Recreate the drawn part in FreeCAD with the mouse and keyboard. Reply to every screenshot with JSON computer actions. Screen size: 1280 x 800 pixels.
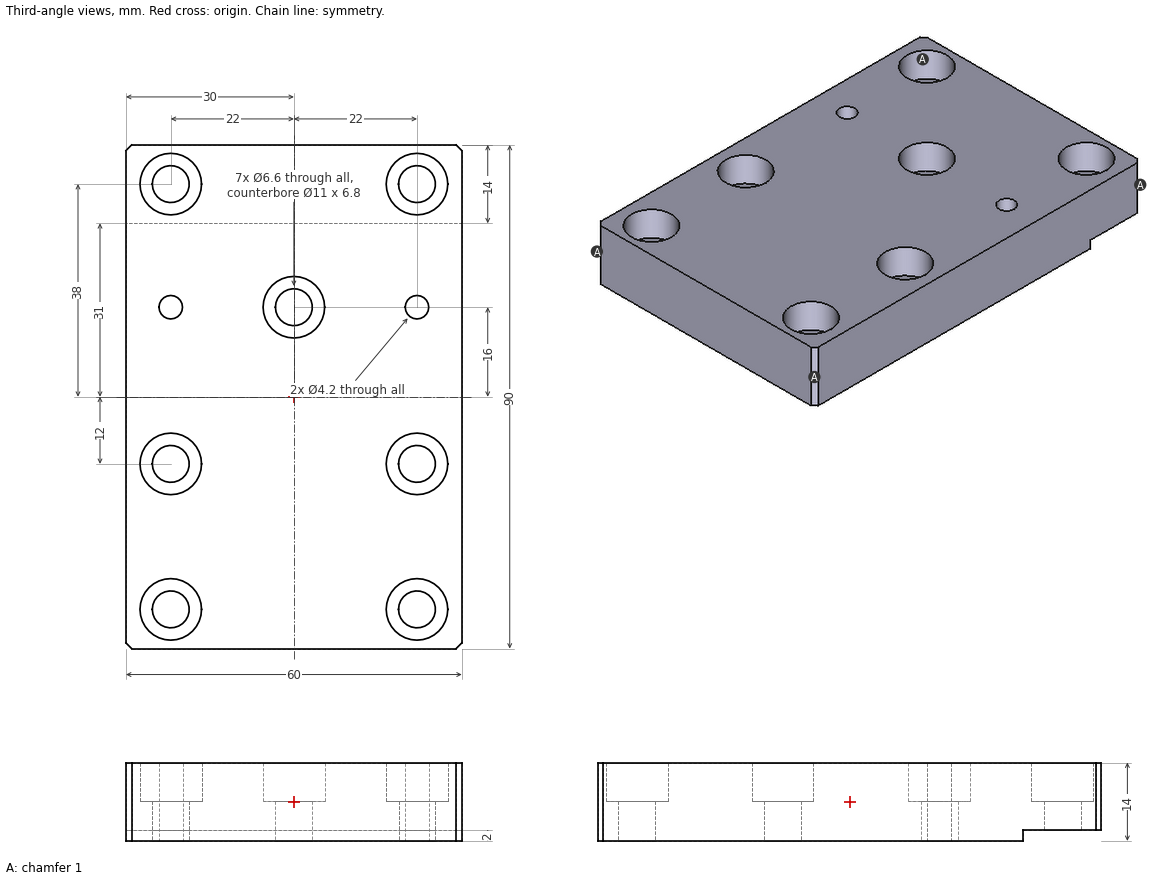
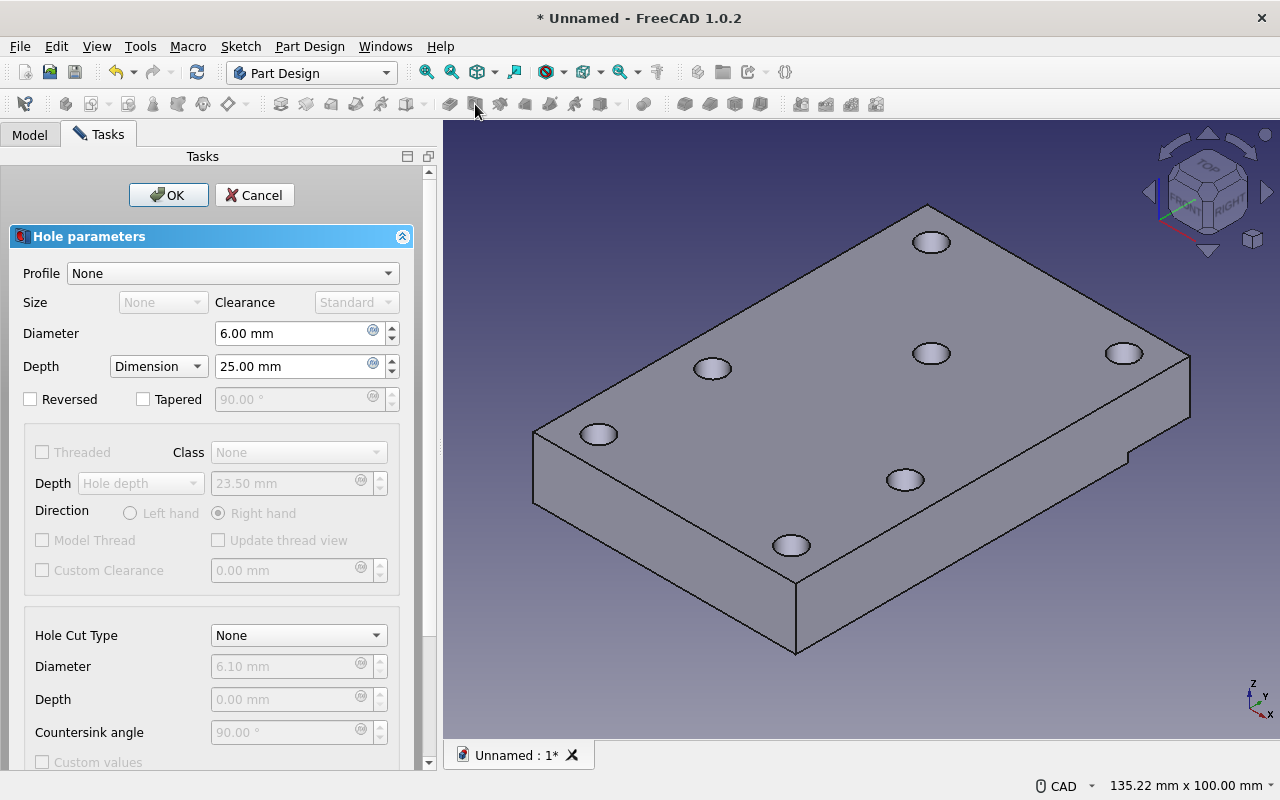
{"action": "triple_click", "coordinate": [300, 334]}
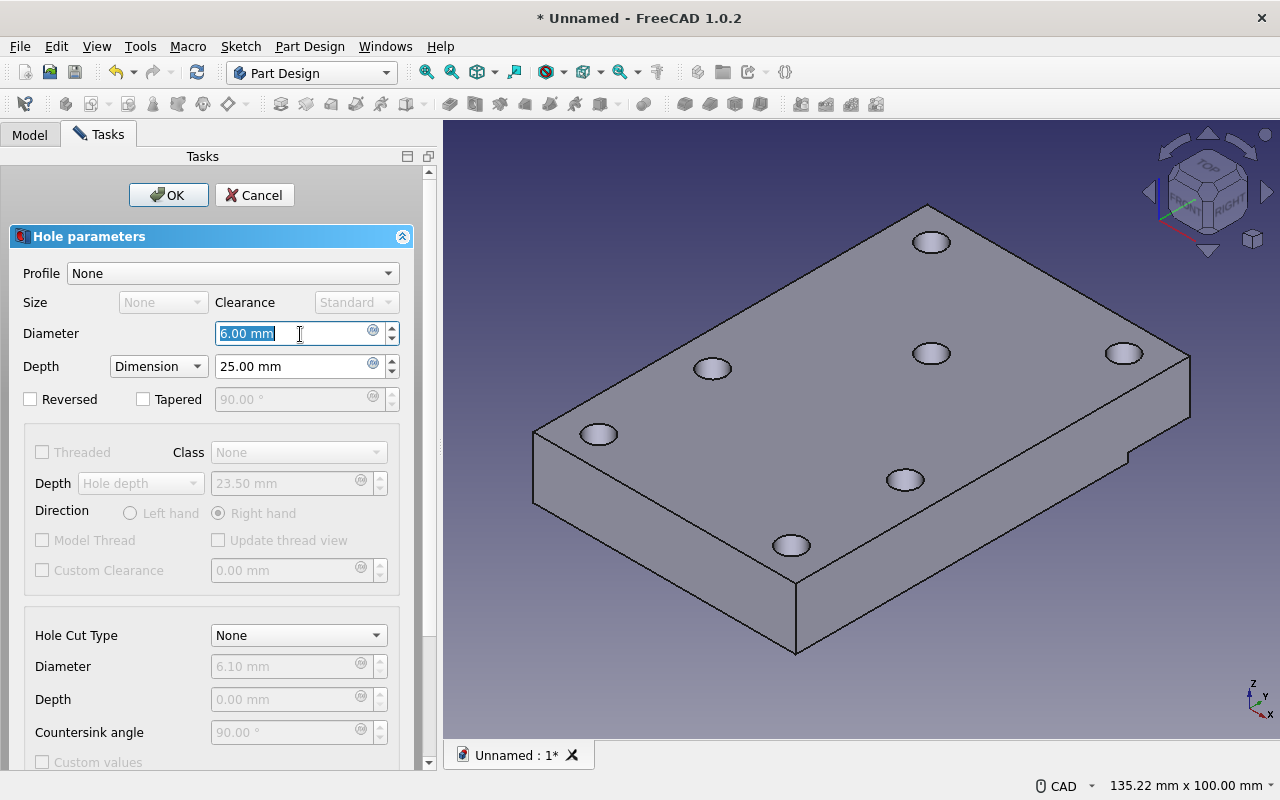
{"action": "type", "text": "6.6"}
{"action": "key", "text": "Tab"}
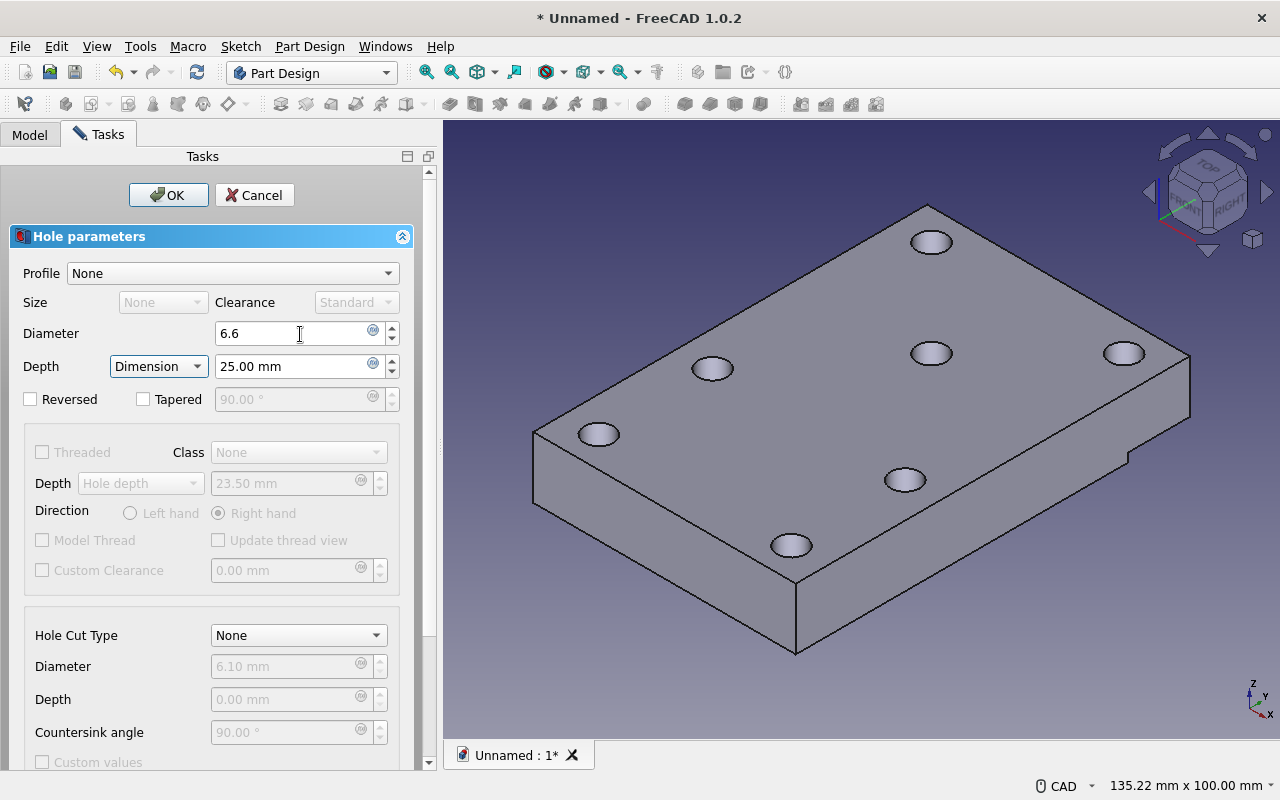
{"action": "left_click", "coordinate": [160, 366]}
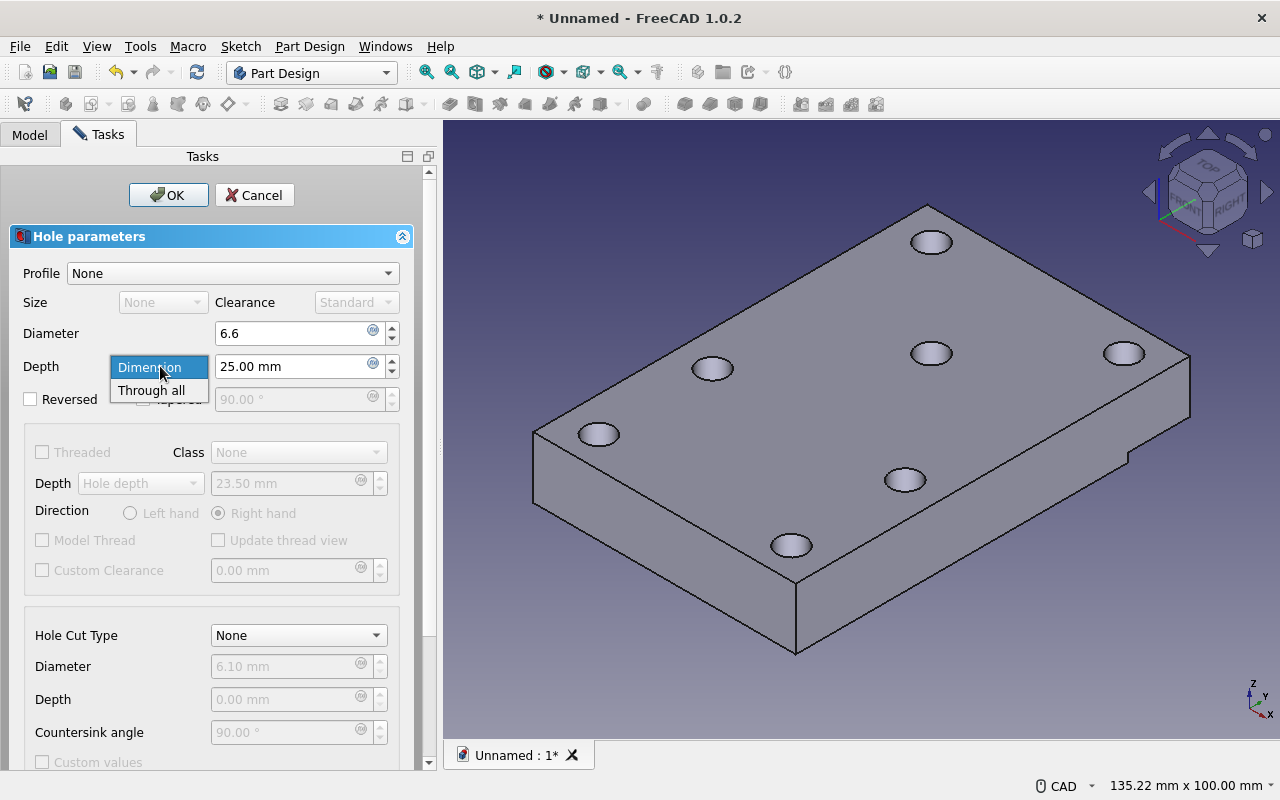
{"action": "left_click", "coordinate": [158, 390]}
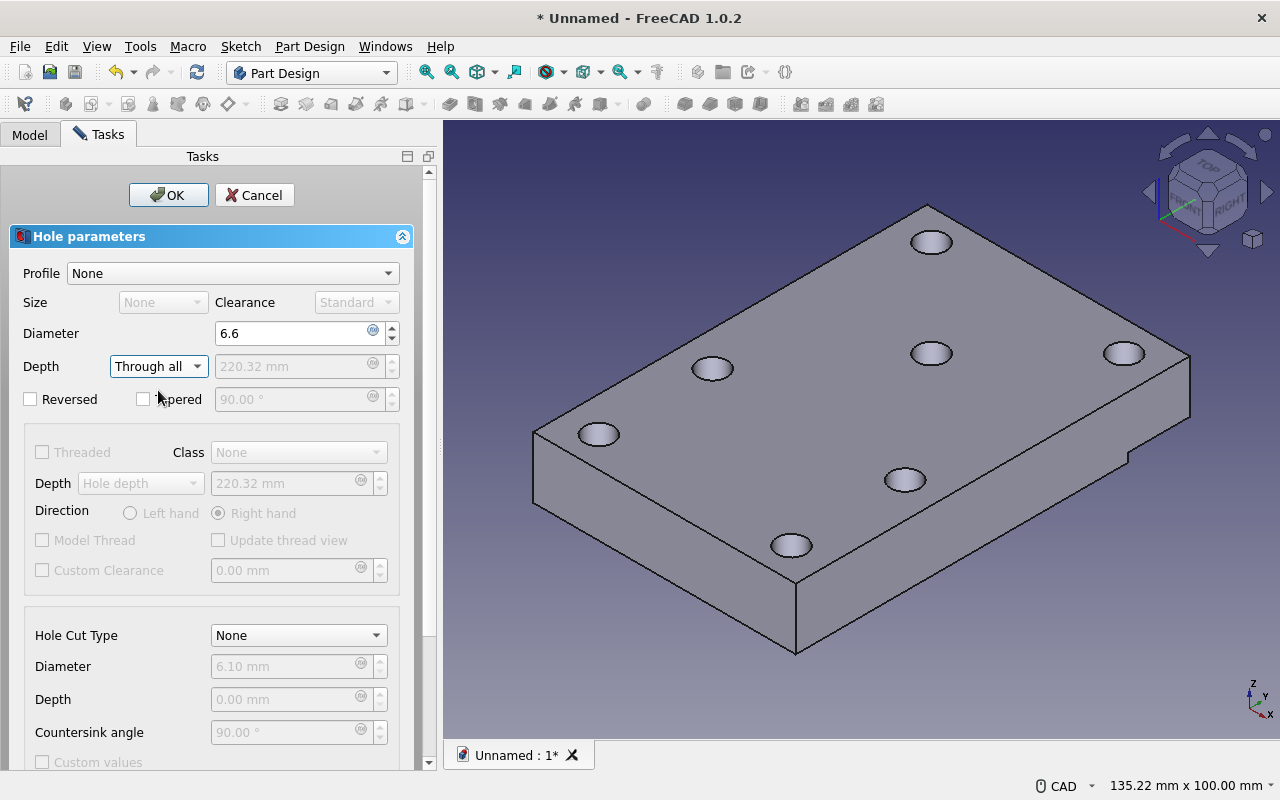
{"action": "left_click", "coordinate": [300, 636]}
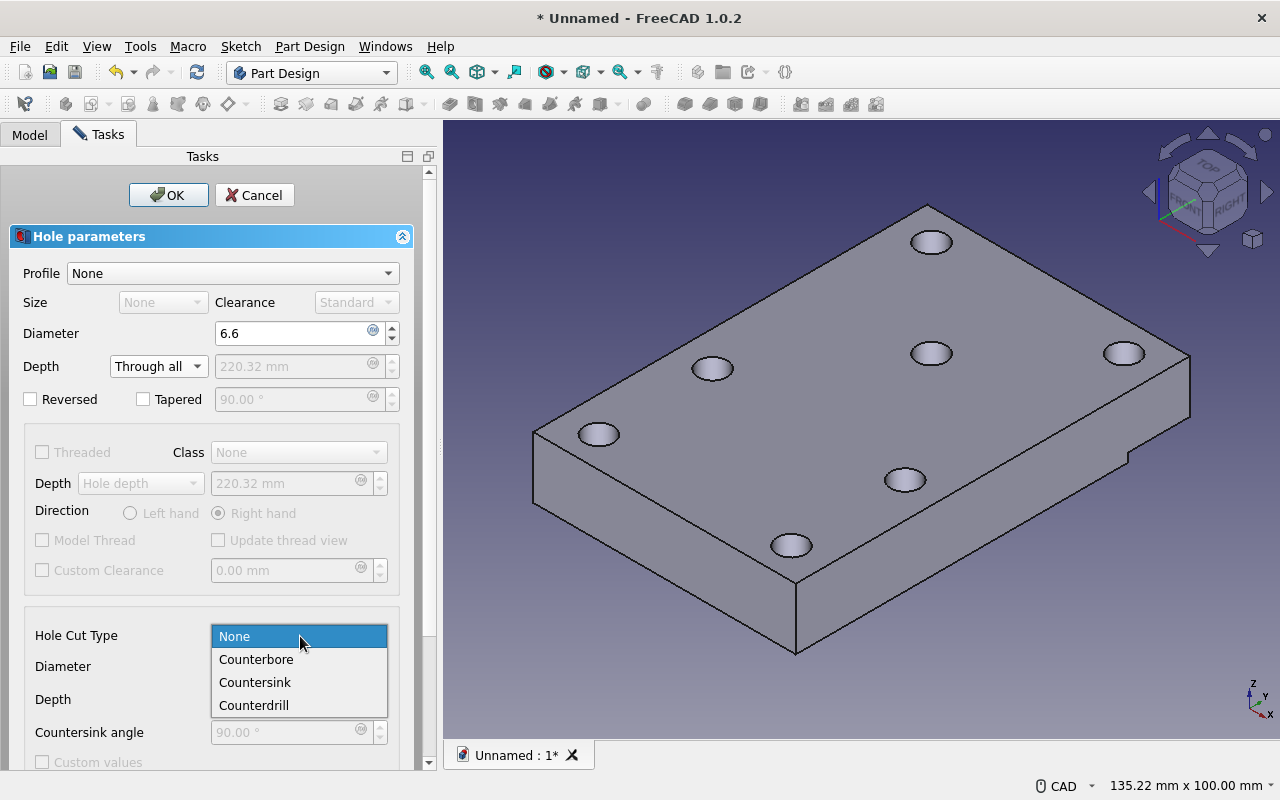
{"action": "left_click", "coordinate": [298, 660]}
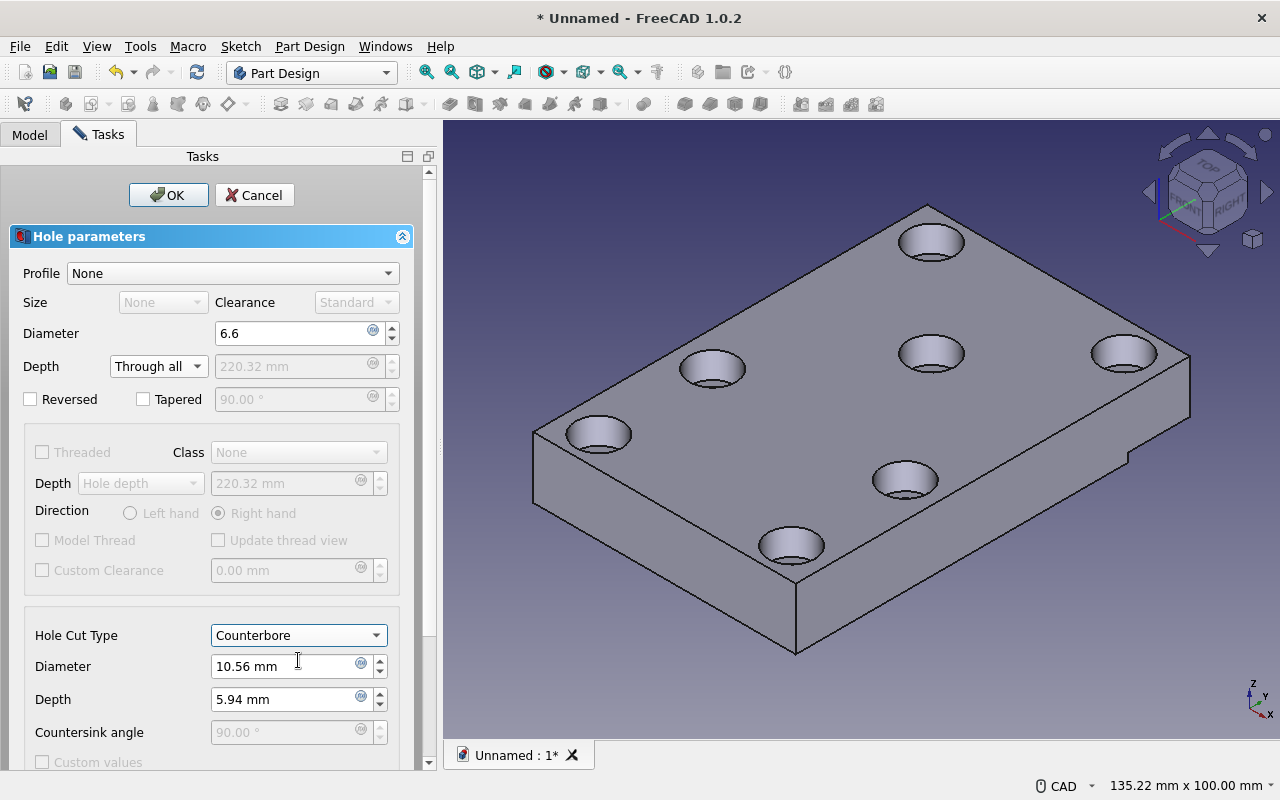
{"action": "triple_click", "coordinate": [292, 666]}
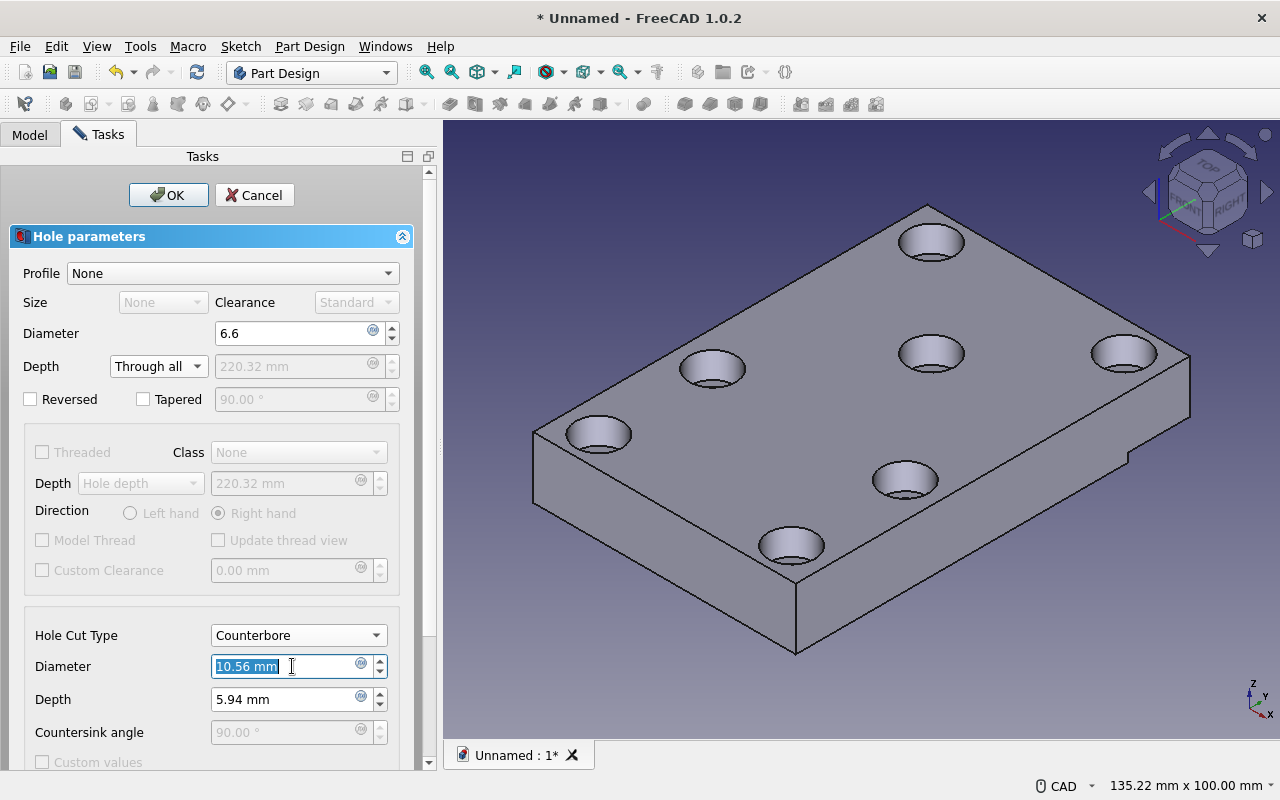
{"action": "type", "text": "11"}
{"action": "key", "text": "Tab"}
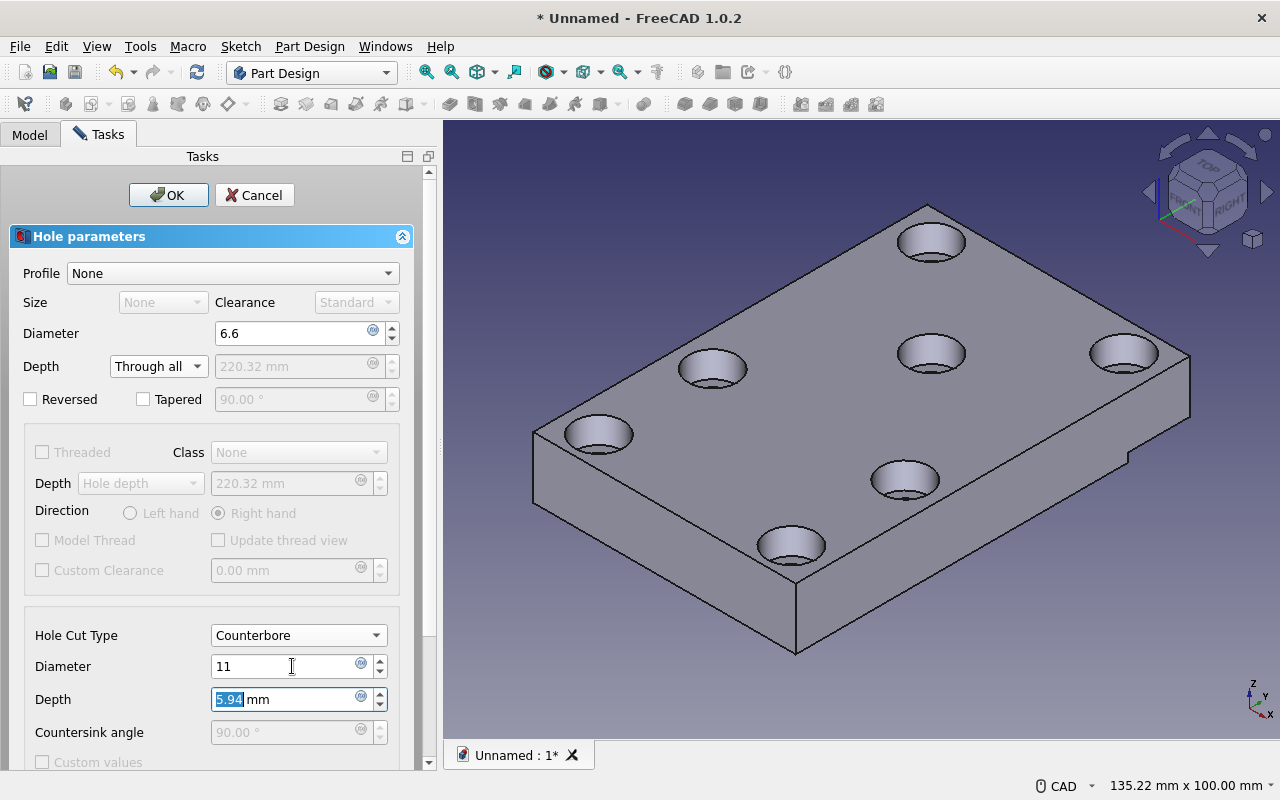
{"action": "type", "text": "6.8"}
{"action": "key", "text": "Tab"}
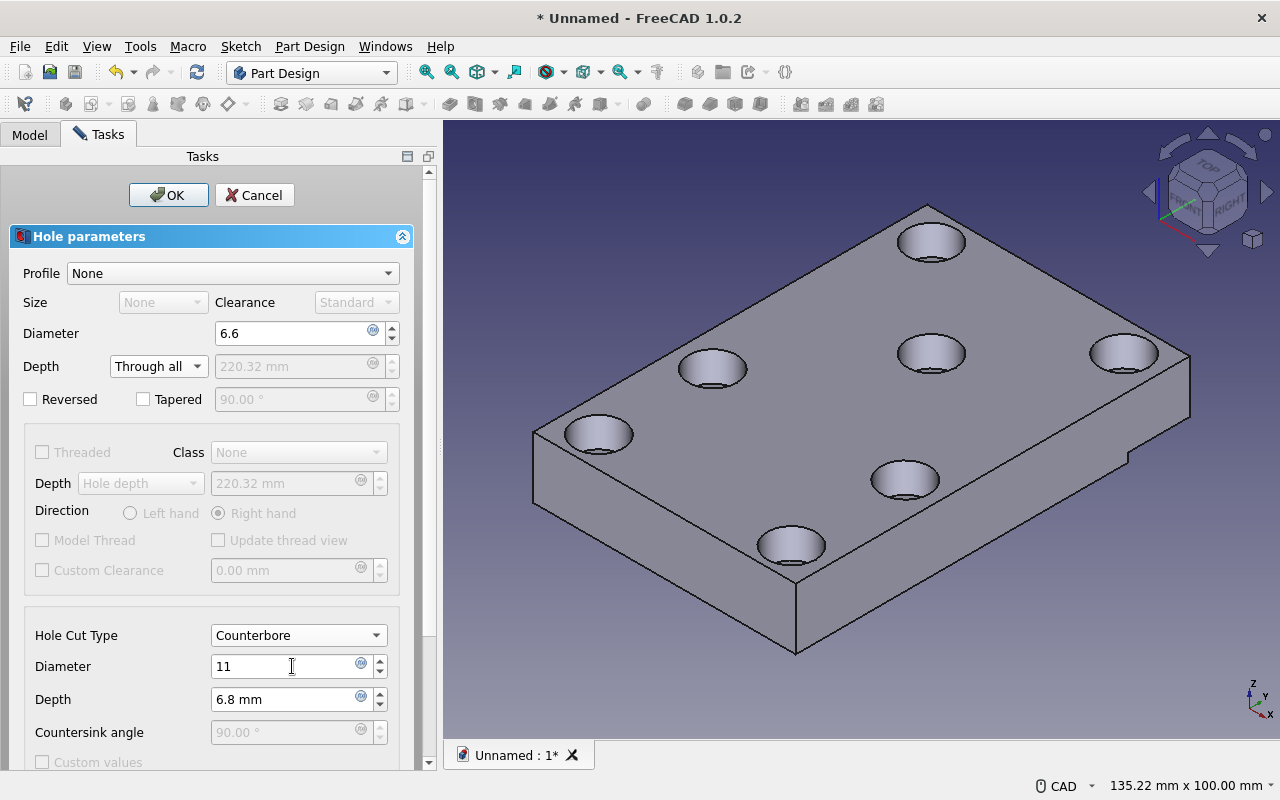
{"action": "left_click", "coordinate": [169, 195]}